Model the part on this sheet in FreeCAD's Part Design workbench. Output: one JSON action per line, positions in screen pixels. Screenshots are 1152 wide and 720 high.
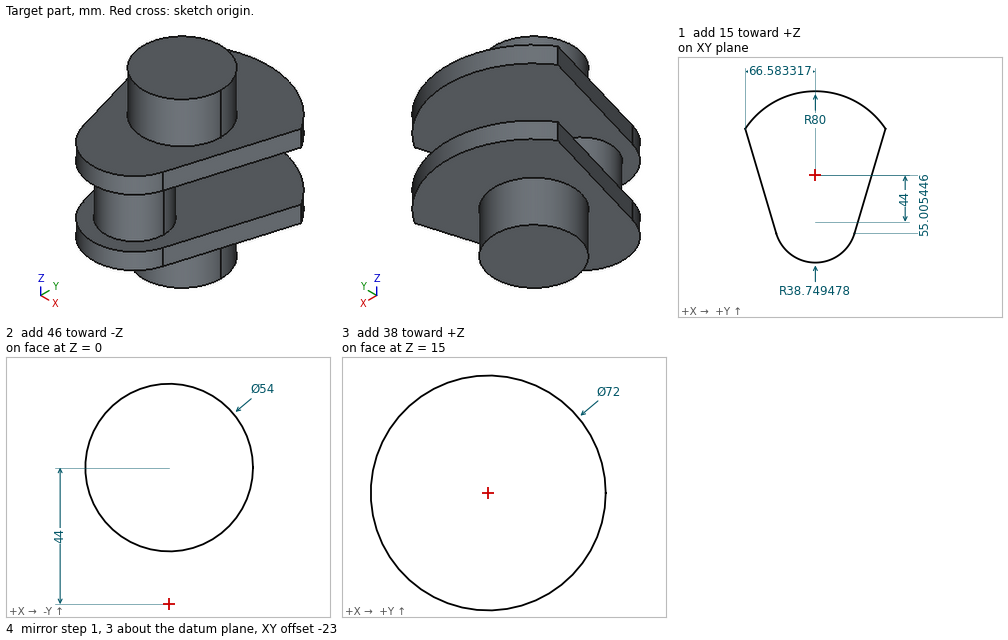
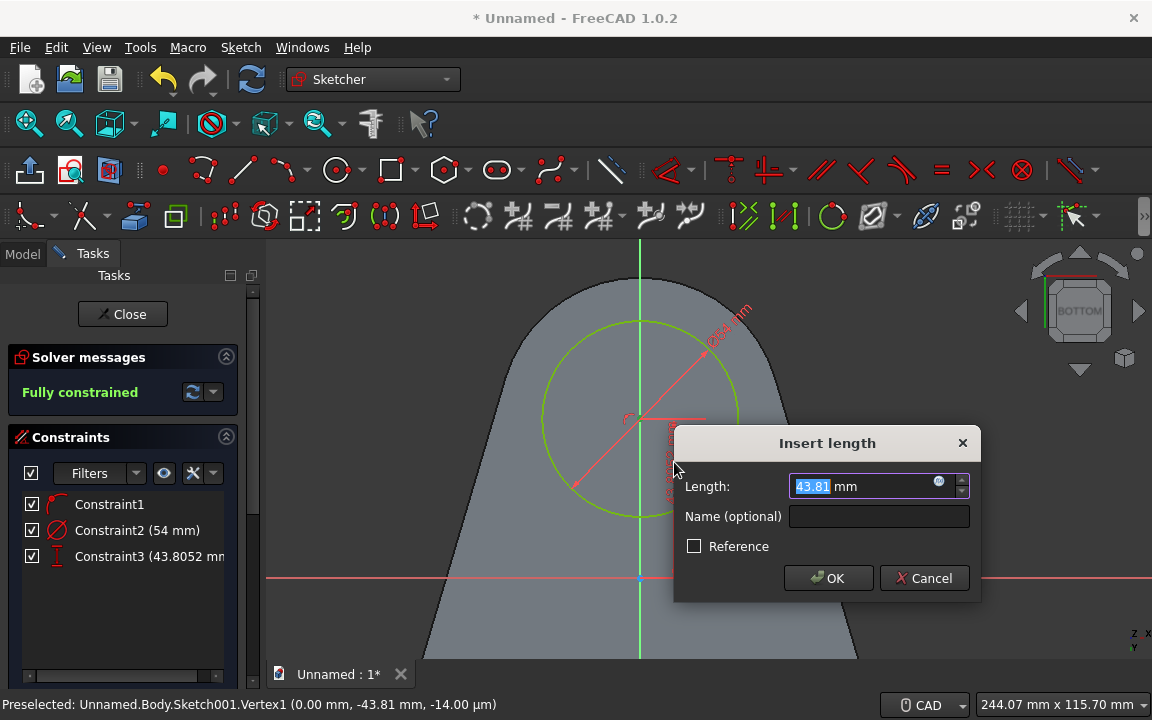
{"action": "type", "text": "44"}
{"action": "key", "text": "Return"}
{"action": "key", "text": "Escape"}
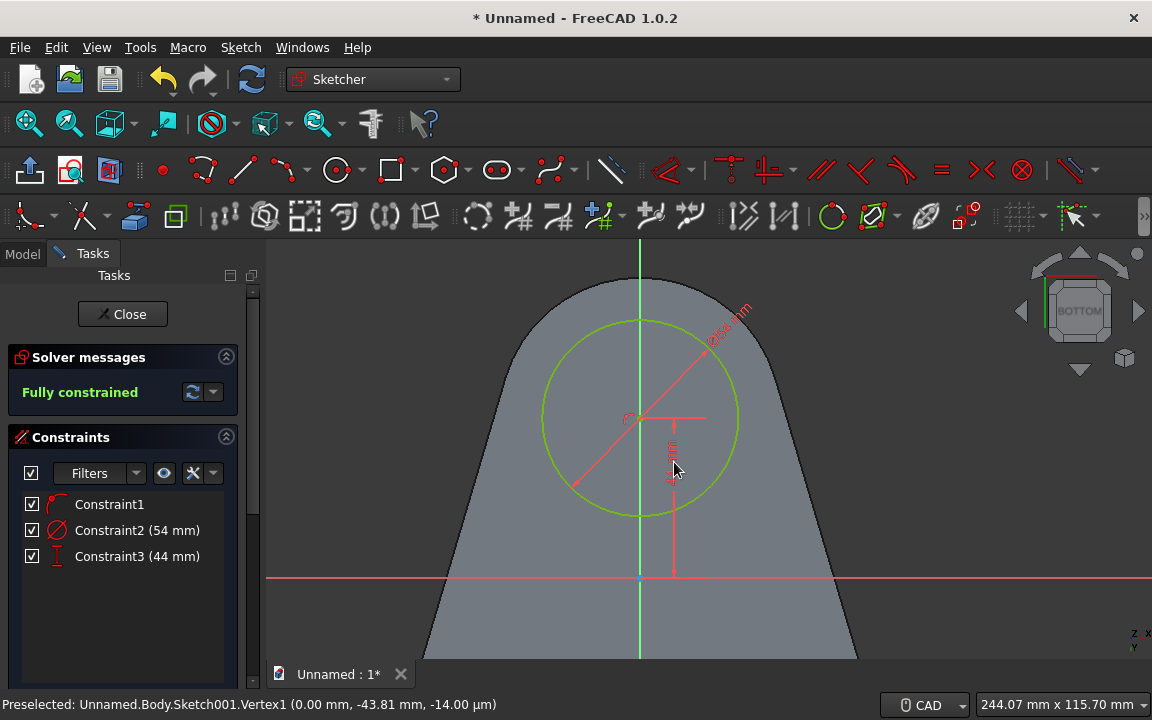
{"action": "left_click", "coordinate": [123, 314]}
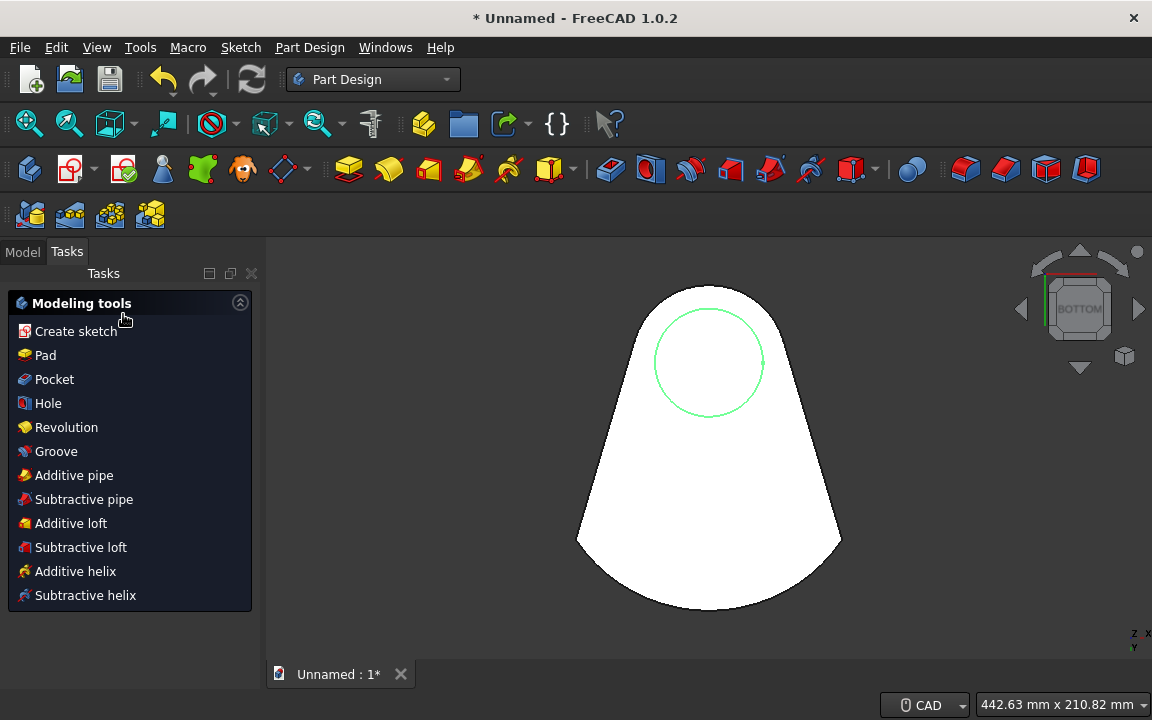
{"action": "left_click", "coordinate": [350, 170]}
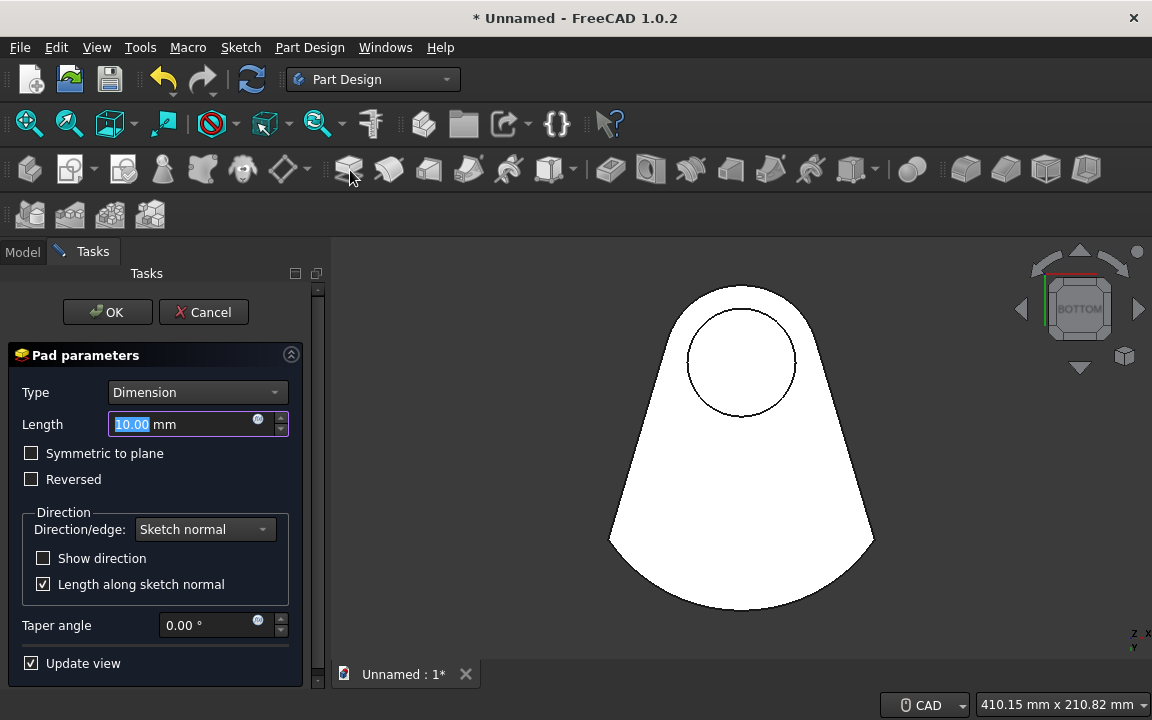
{"action": "type", "text": "46"}
{"action": "key", "text": "Tab"}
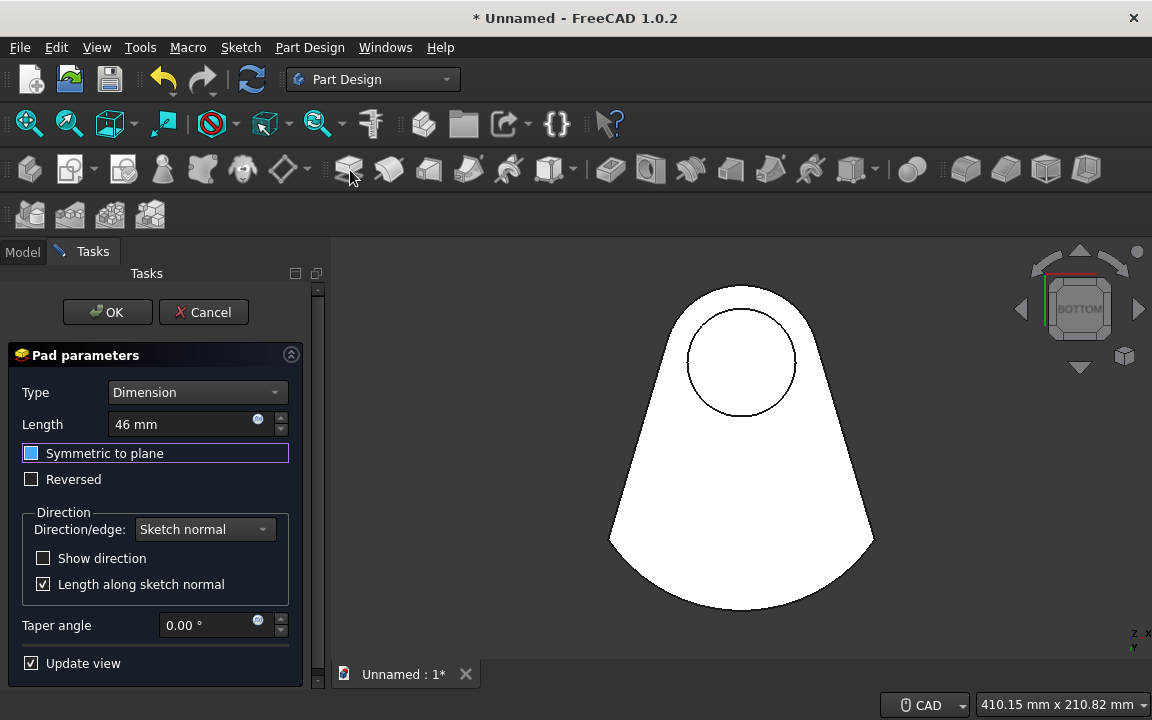
{"action": "left_click", "coordinate": [108, 312]}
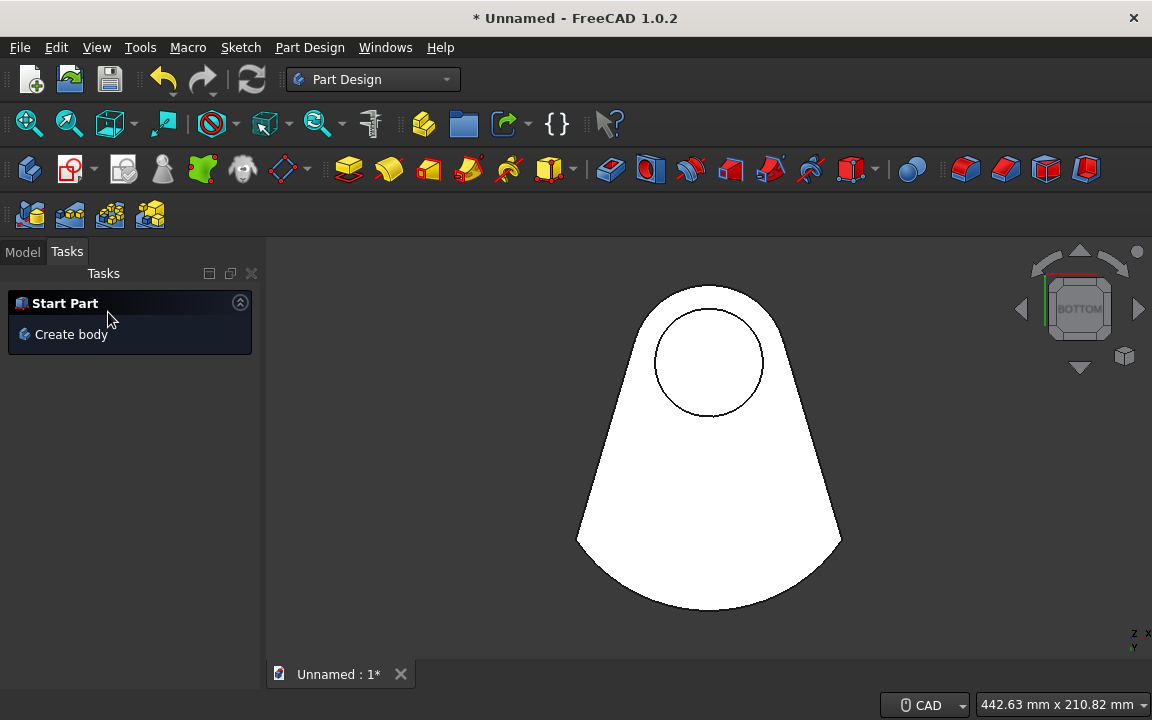
{"action": "key", "text": "0"}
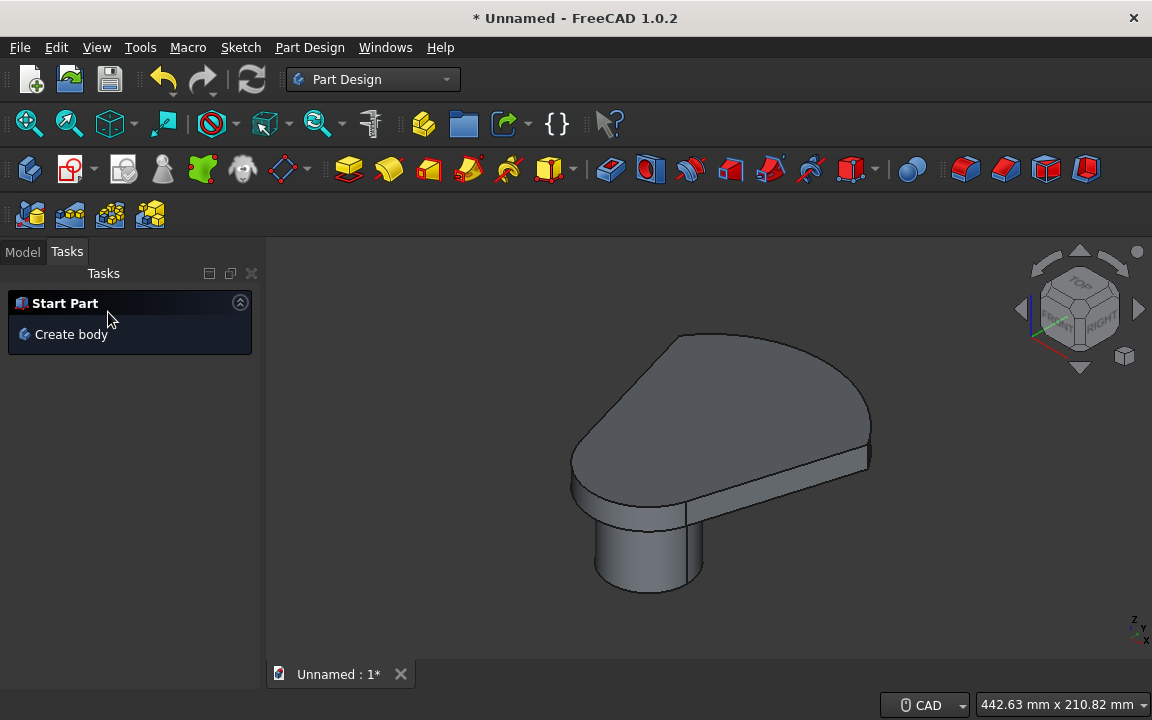
{"action": "left_click", "coordinate": [742, 408]}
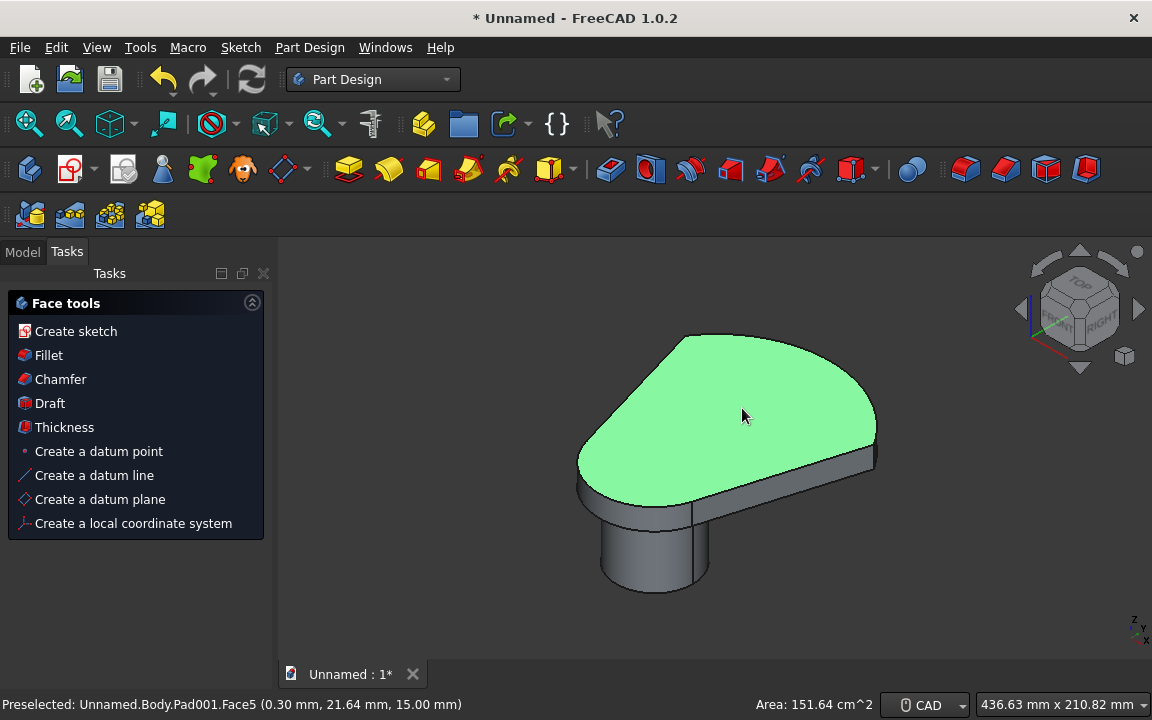
{"action": "left_click", "coordinate": [70, 170]}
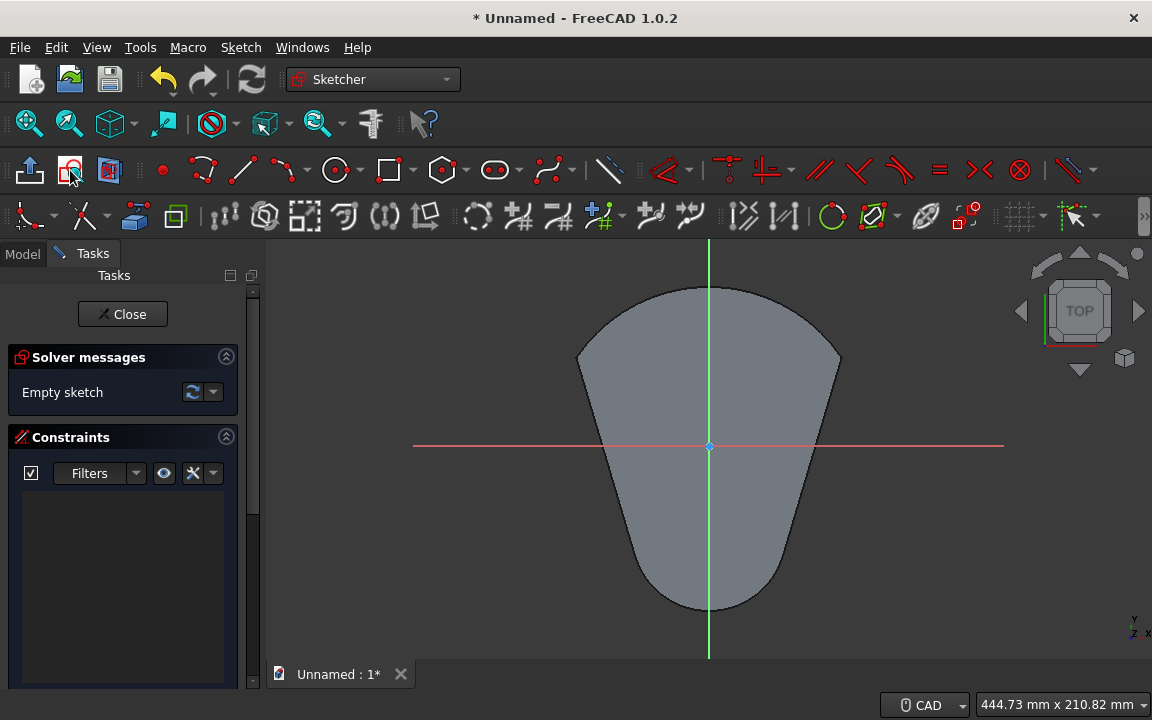
{"action": "scroll", "coordinate": [792, 443], "scroll_direction": "up", "scroll_amount": 3}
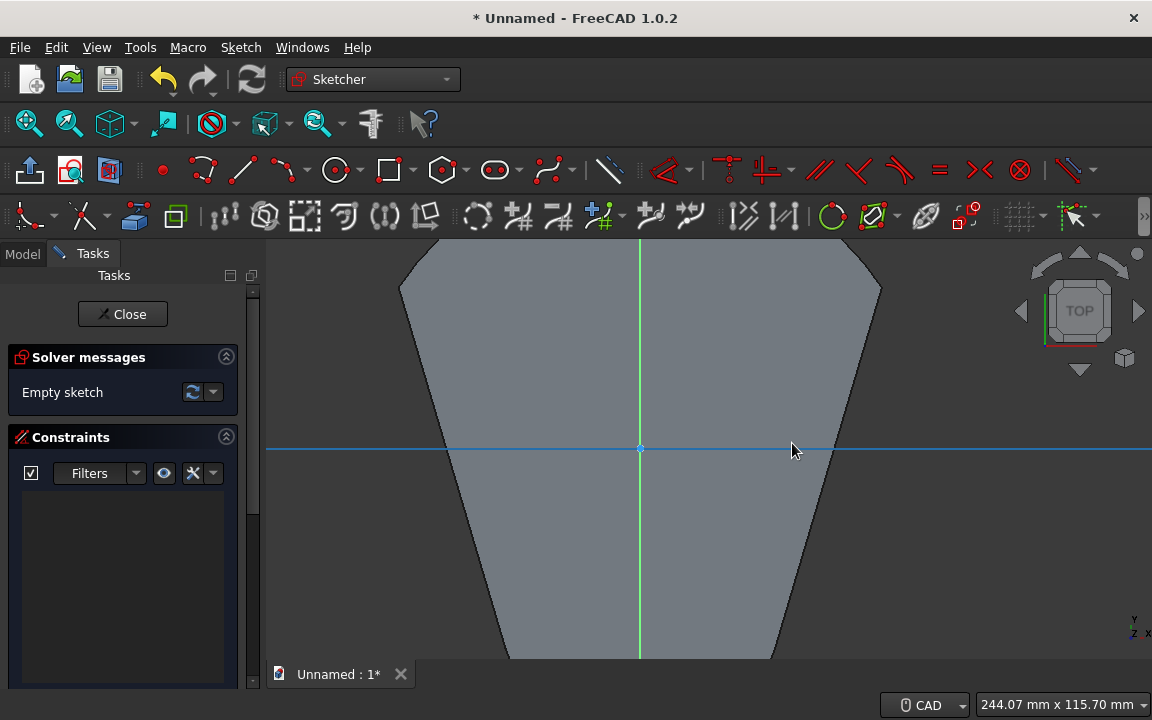
{"action": "key", "text": "g c"}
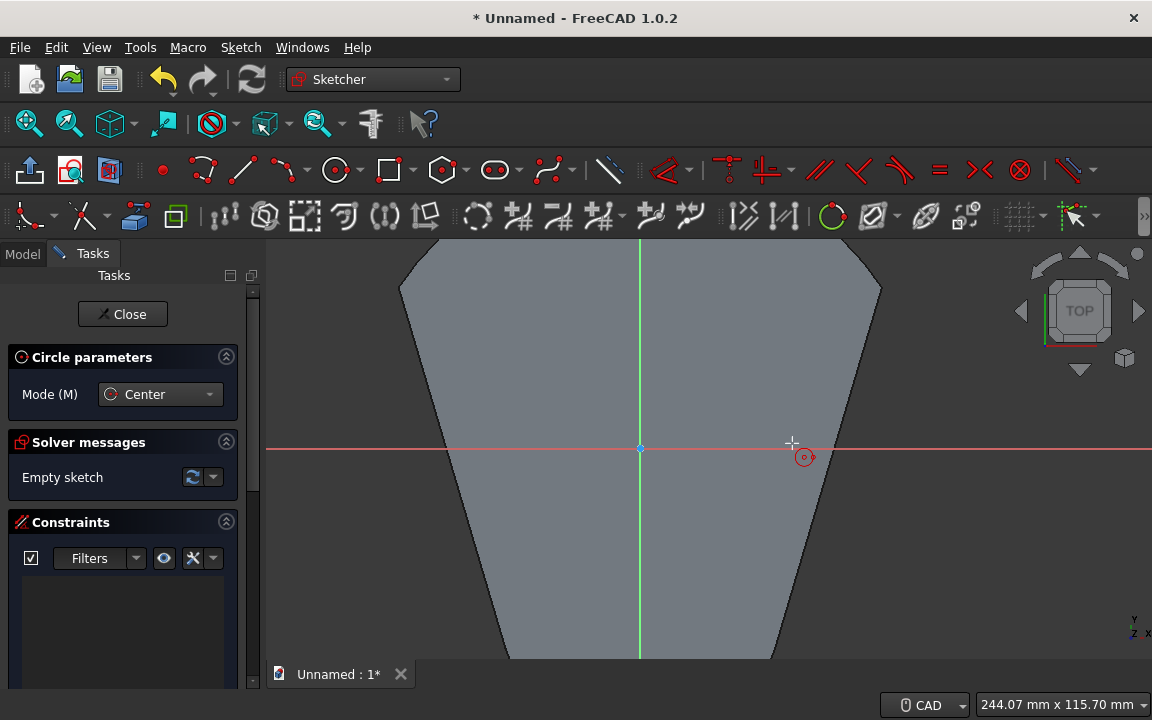
{"action": "left_click", "coordinate": [640, 449]}
{"action": "left_click", "coordinate": [733, 356]}
{"action": "key", "text": "Escape"}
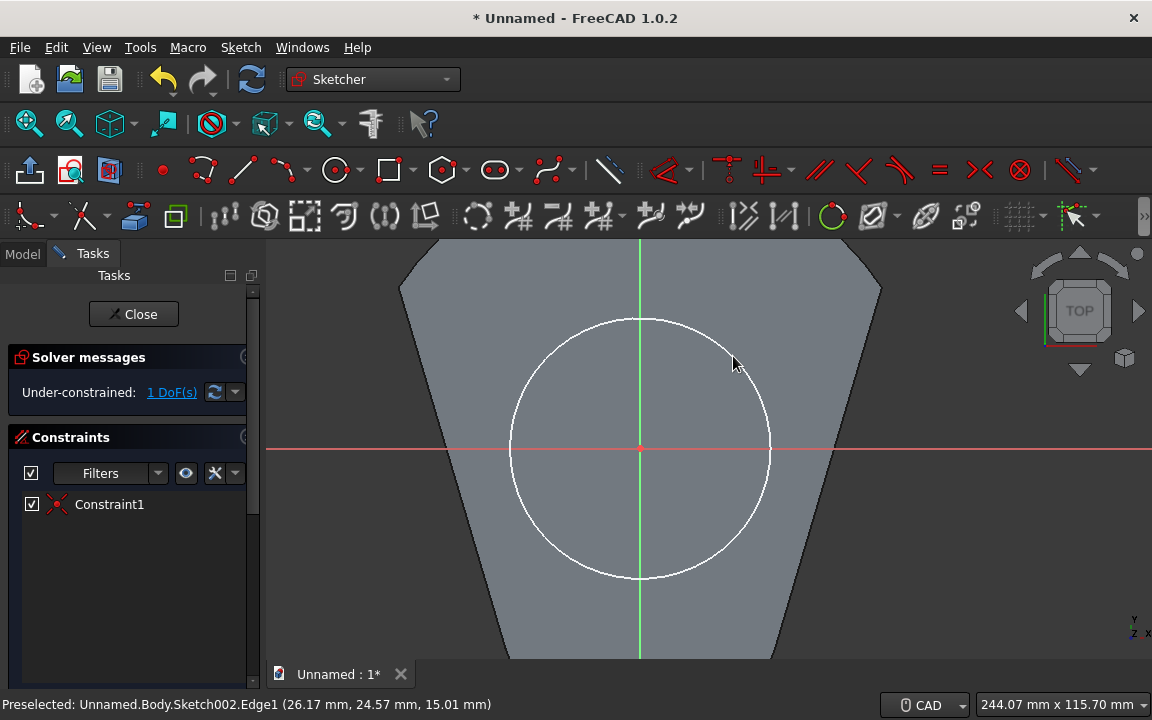
{"action": "key", "text": "d"}